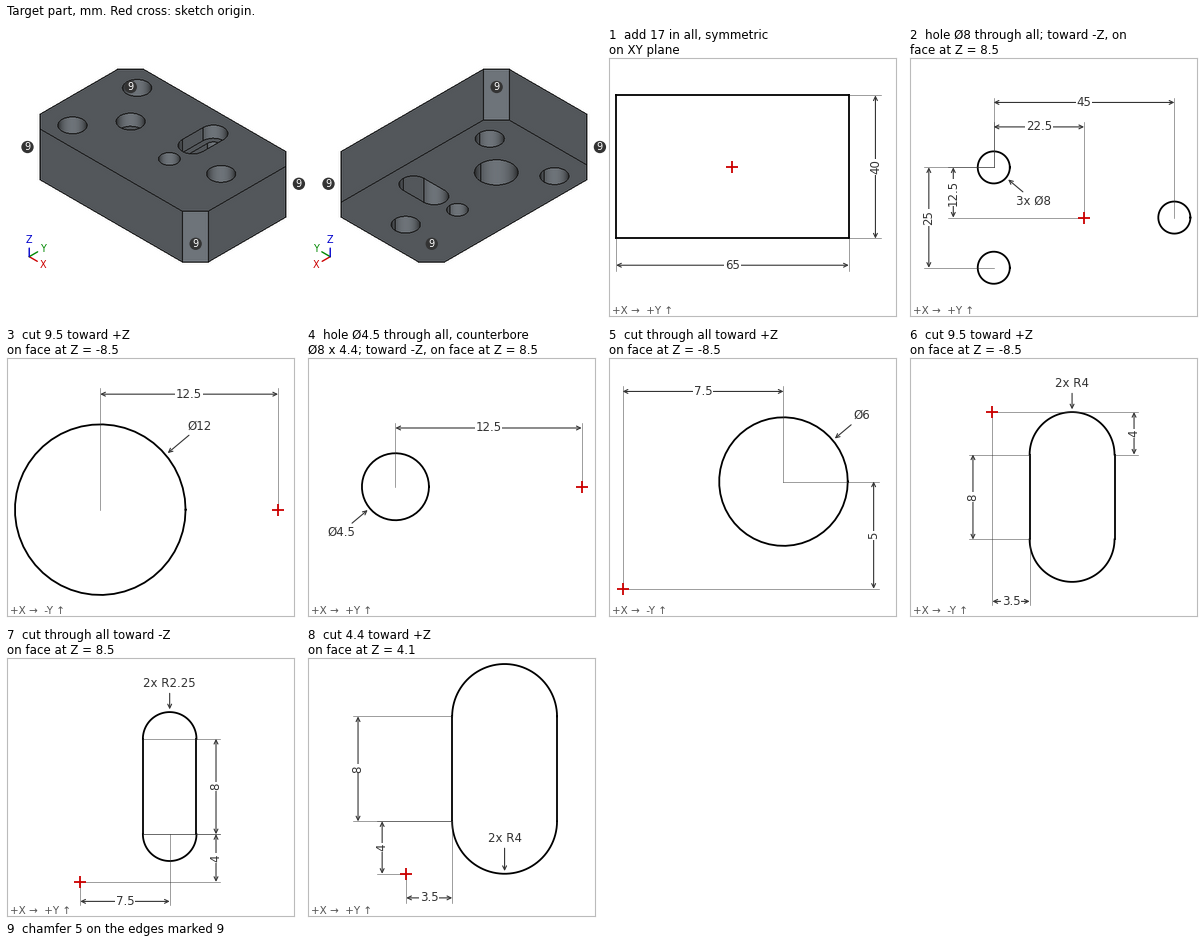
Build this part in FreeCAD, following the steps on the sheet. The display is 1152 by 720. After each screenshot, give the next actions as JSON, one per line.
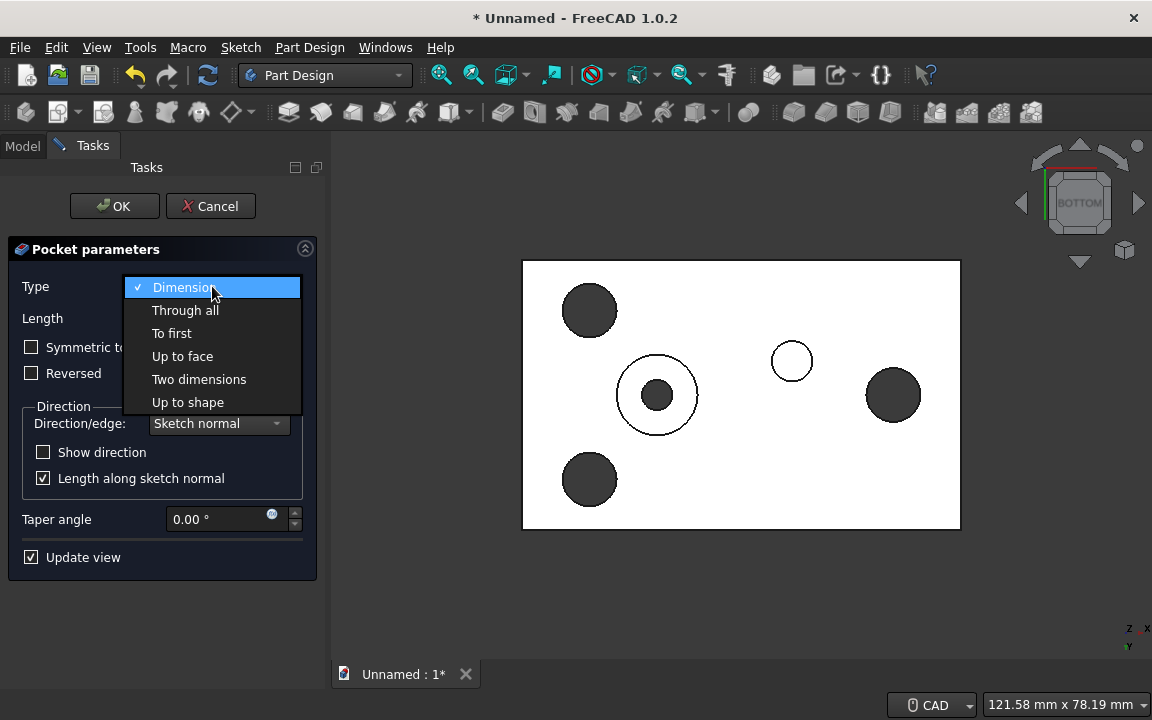
{"action": "left_click", "coordinate": [212, 310]}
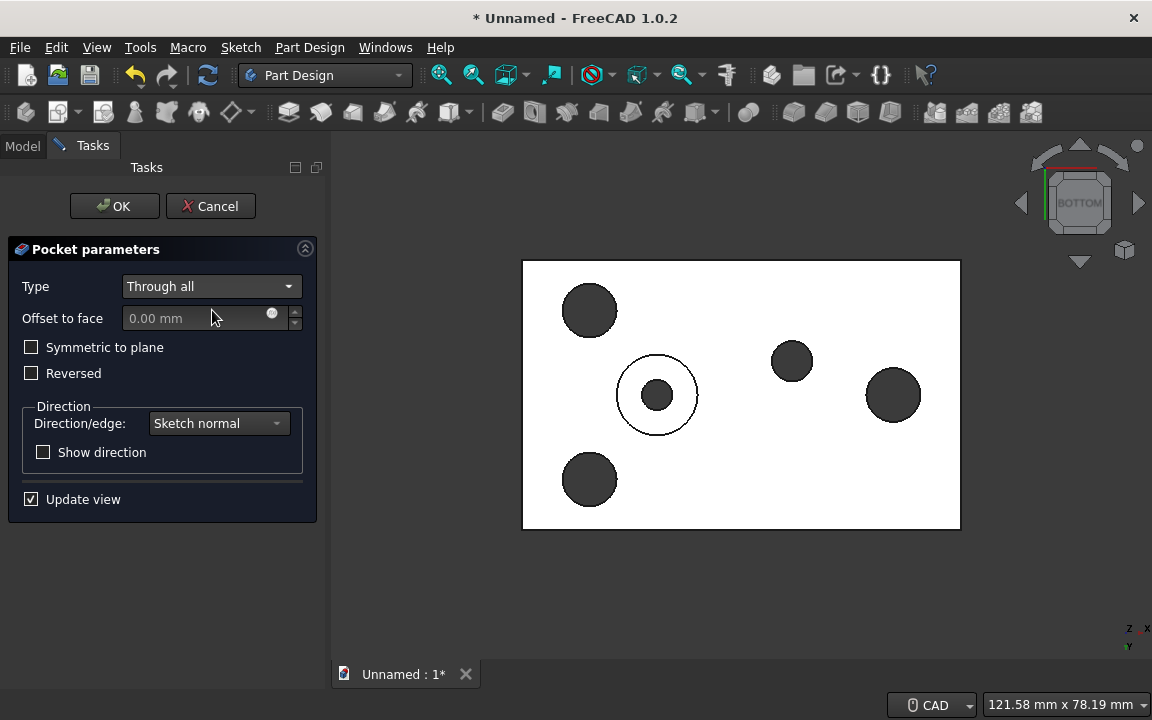
{"action": "left_click", "coordinate": [115, 206]}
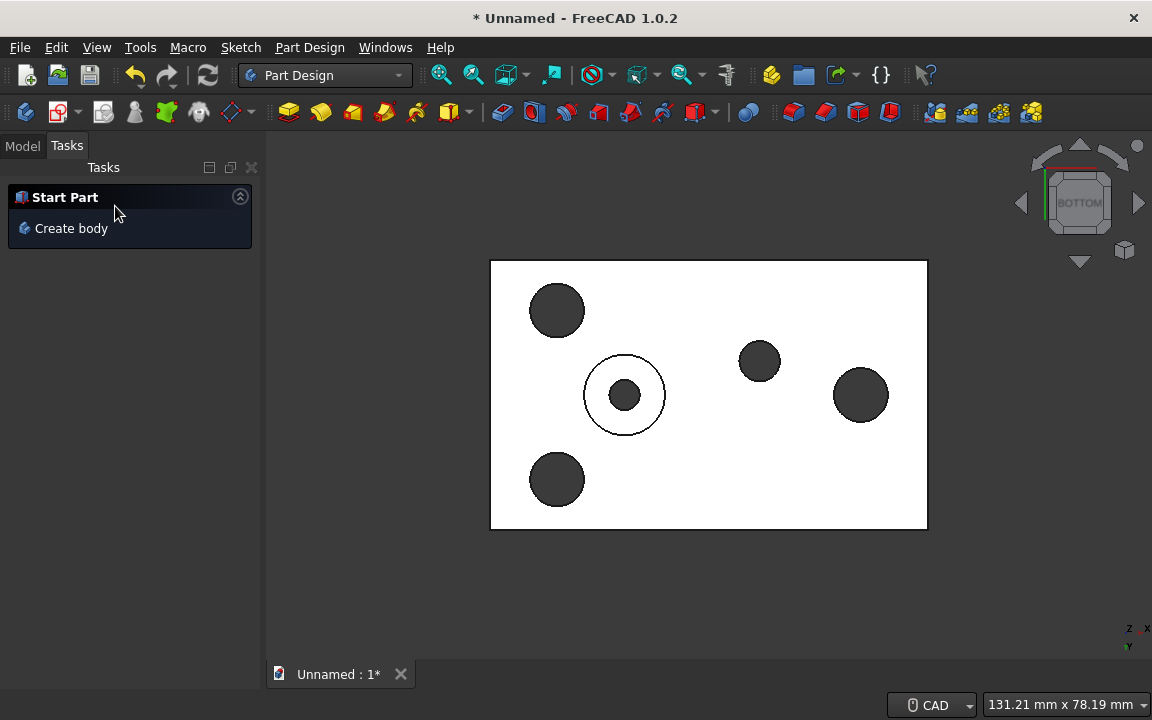
{"action": "left_click", "coordinate": [772, 471]}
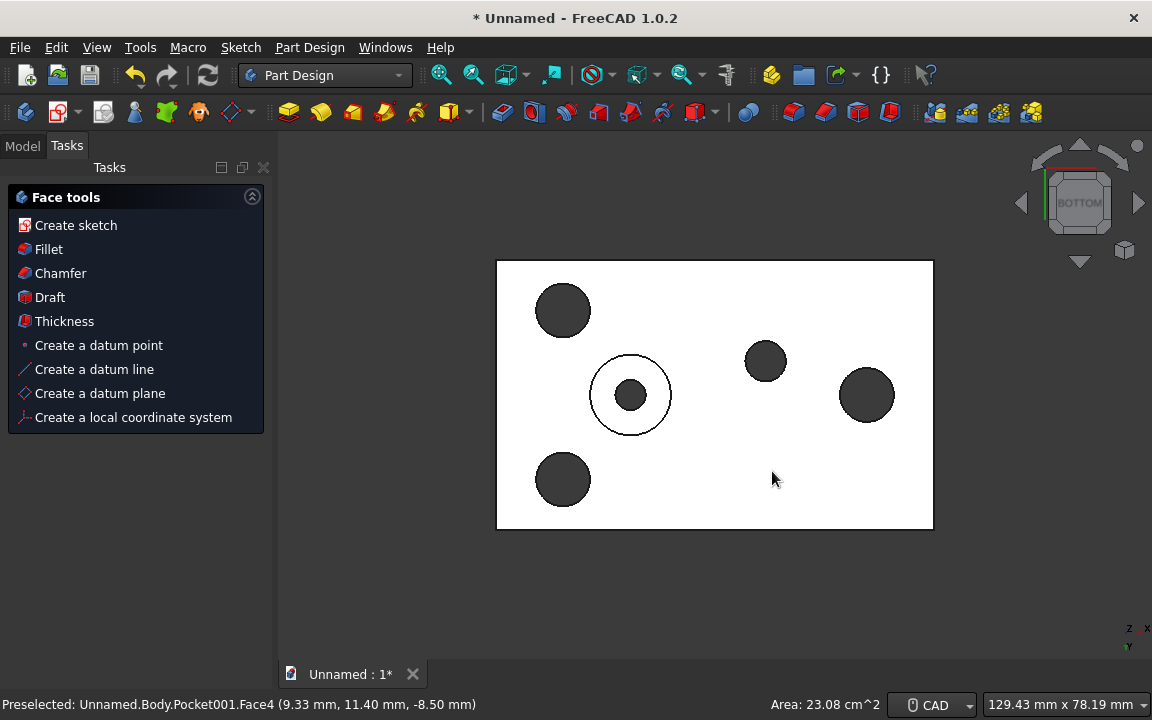
{"action": "left_click", "coordinate": [58, 112]}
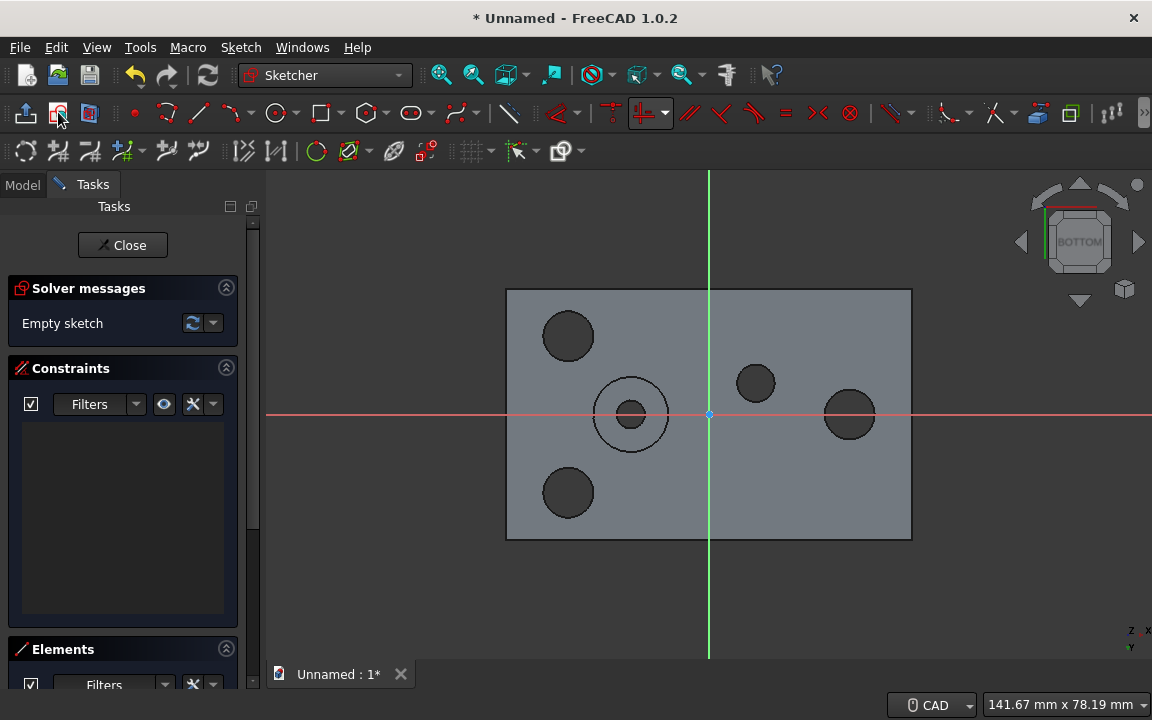
{"action": "scroll", "coordinate": [790, 486], "scroll_direction": "up", "scroll_amount": 6}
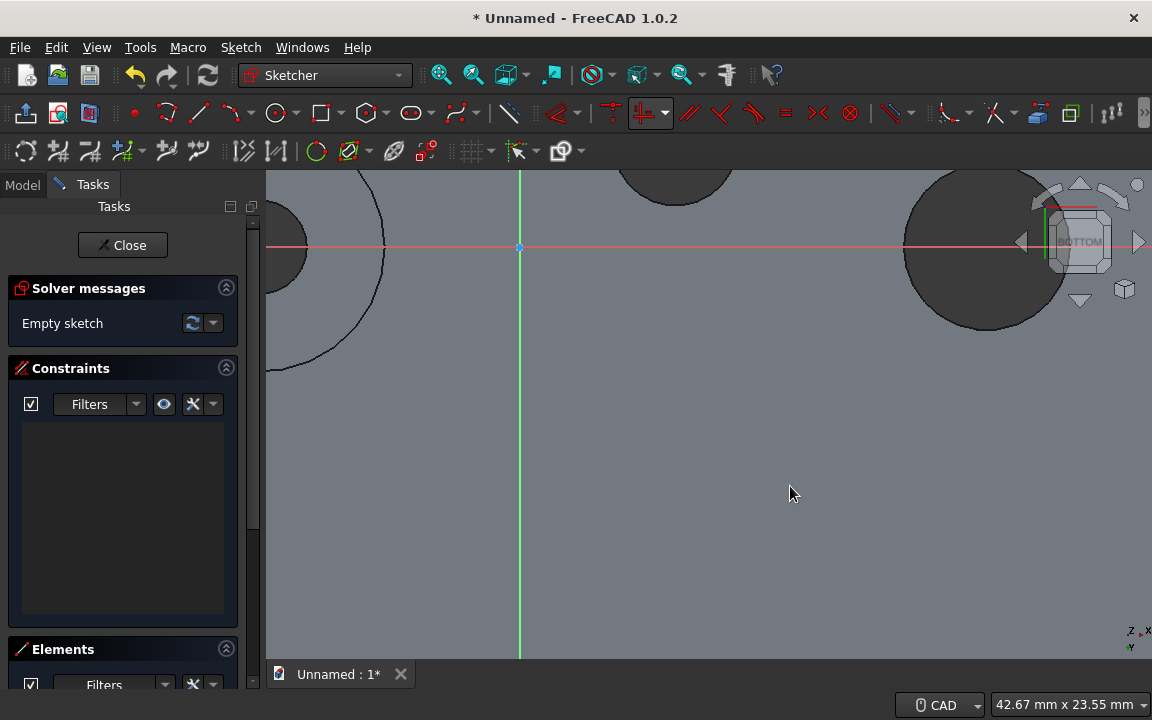
{"action": "left_click", "coordinate": [412, 114]}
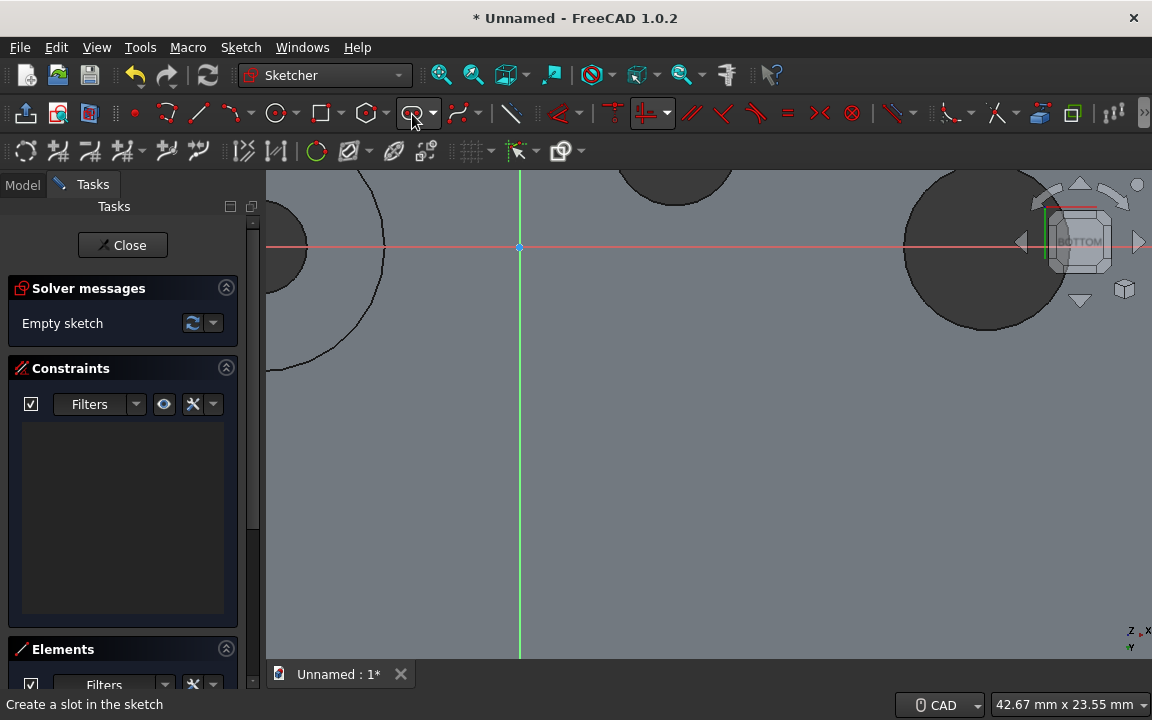
{"action": "left_click", "coordinate": [675, 496]}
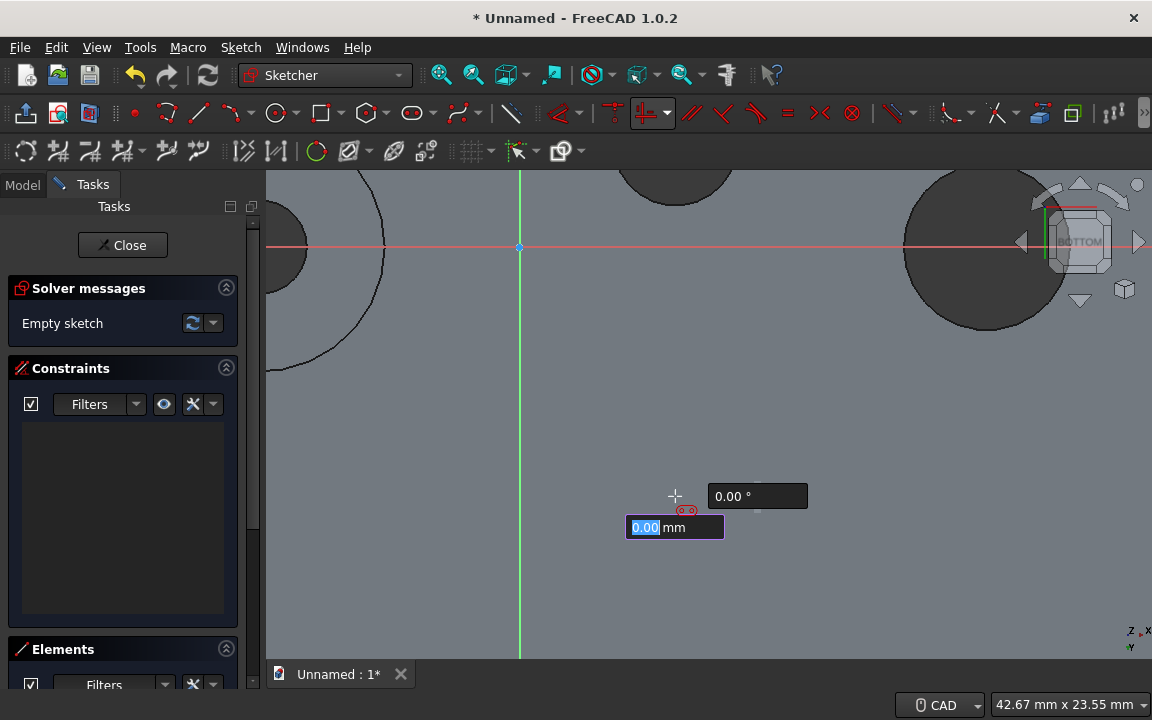
{"action": "left_click", "coordinate": [675, 330]}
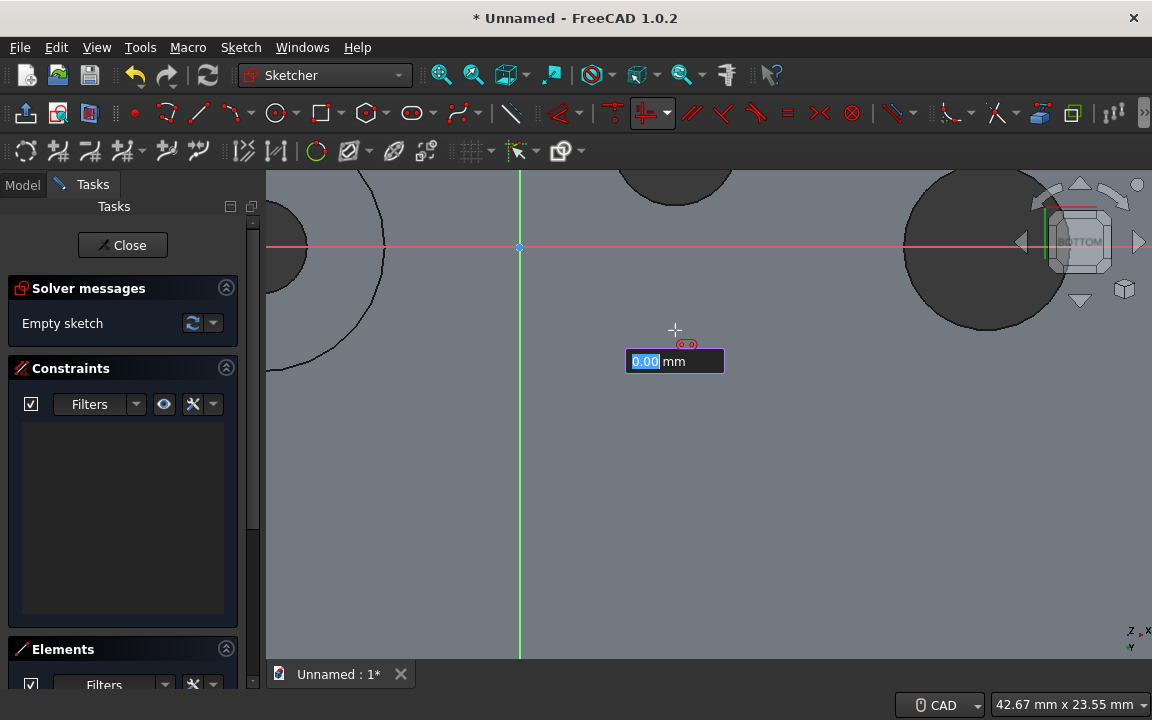
{"action": "left_click", "coordinate": [758, 413]}
{"action": "key", "text": "Escape"}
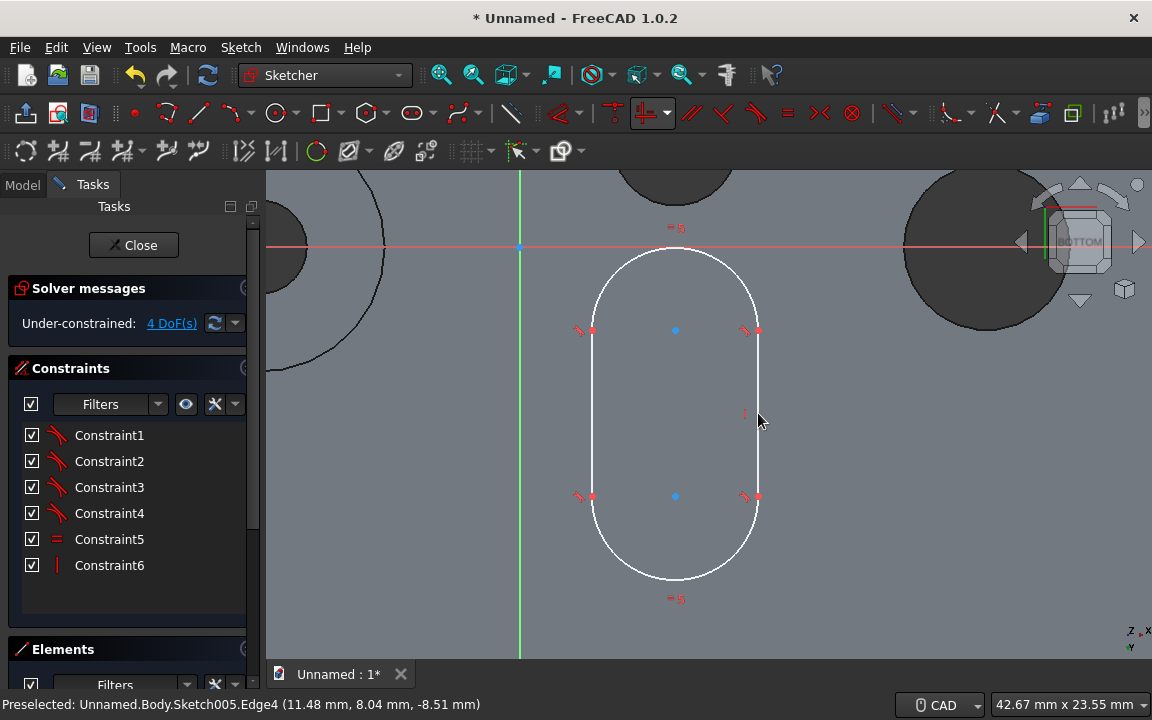
{"action": "left_click", "coordinate": [558, 114]}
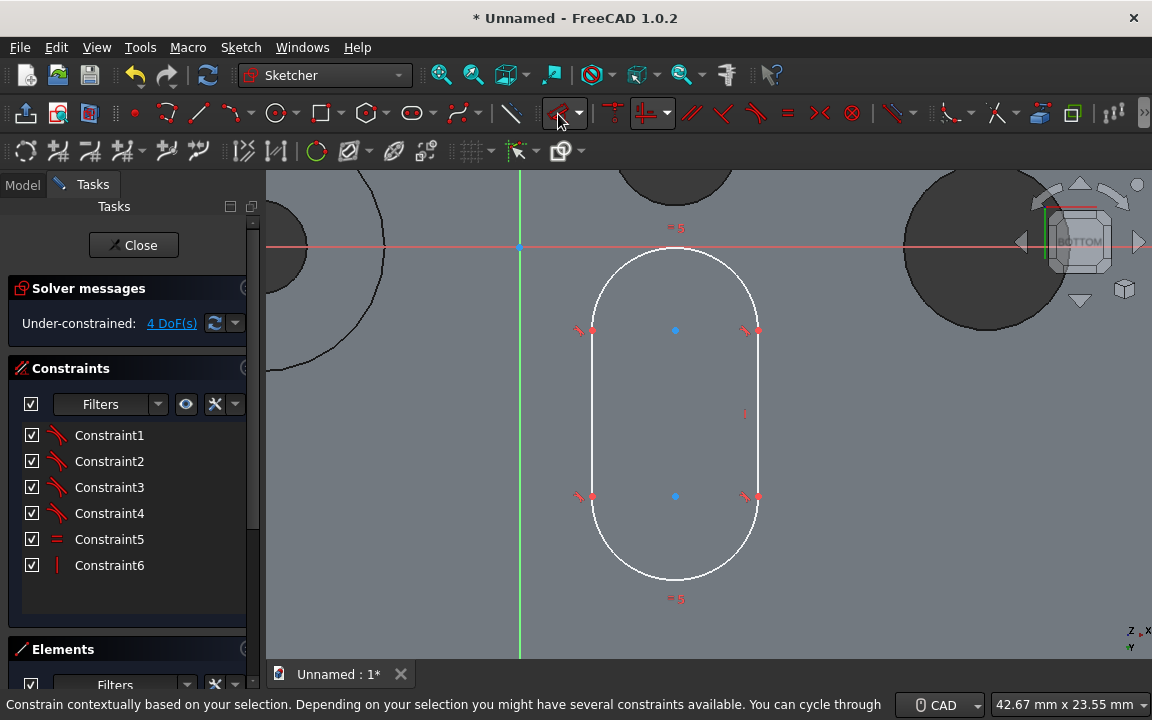
{"action": "left_click", "coordinate": [626, 564]}
{"action": "left_click", "coordinate": [607, 590]}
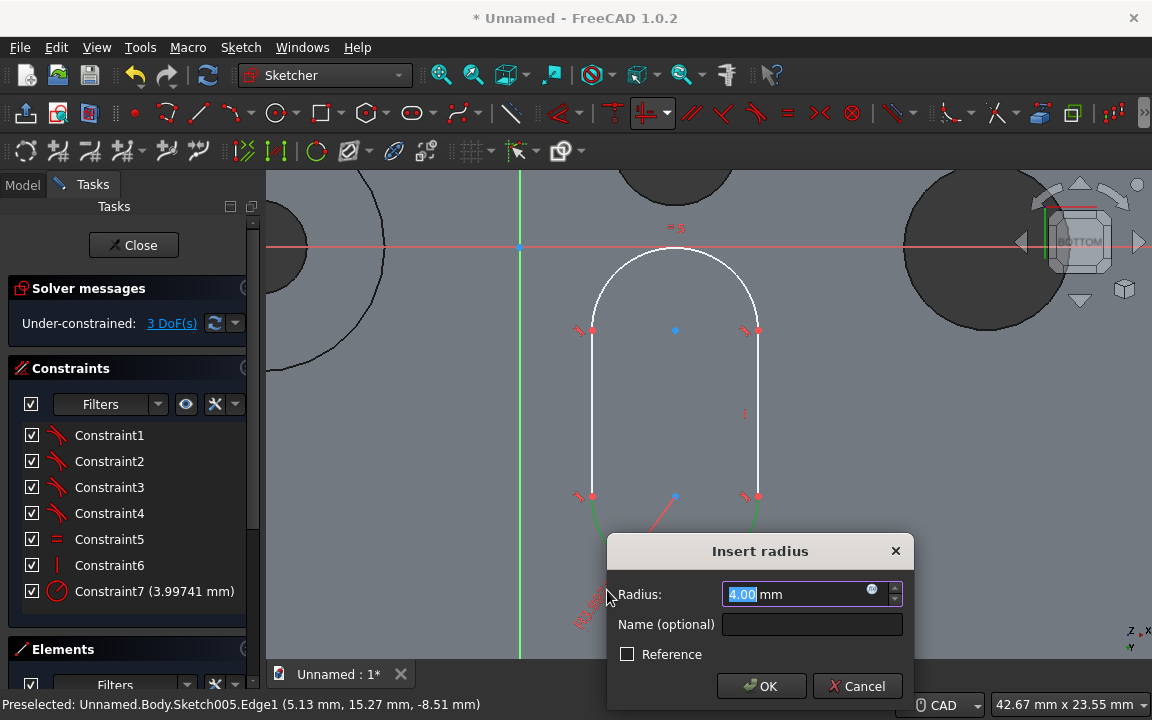
{"action": "type", "text": "4"}
{"action": "key", "text": "Return"}